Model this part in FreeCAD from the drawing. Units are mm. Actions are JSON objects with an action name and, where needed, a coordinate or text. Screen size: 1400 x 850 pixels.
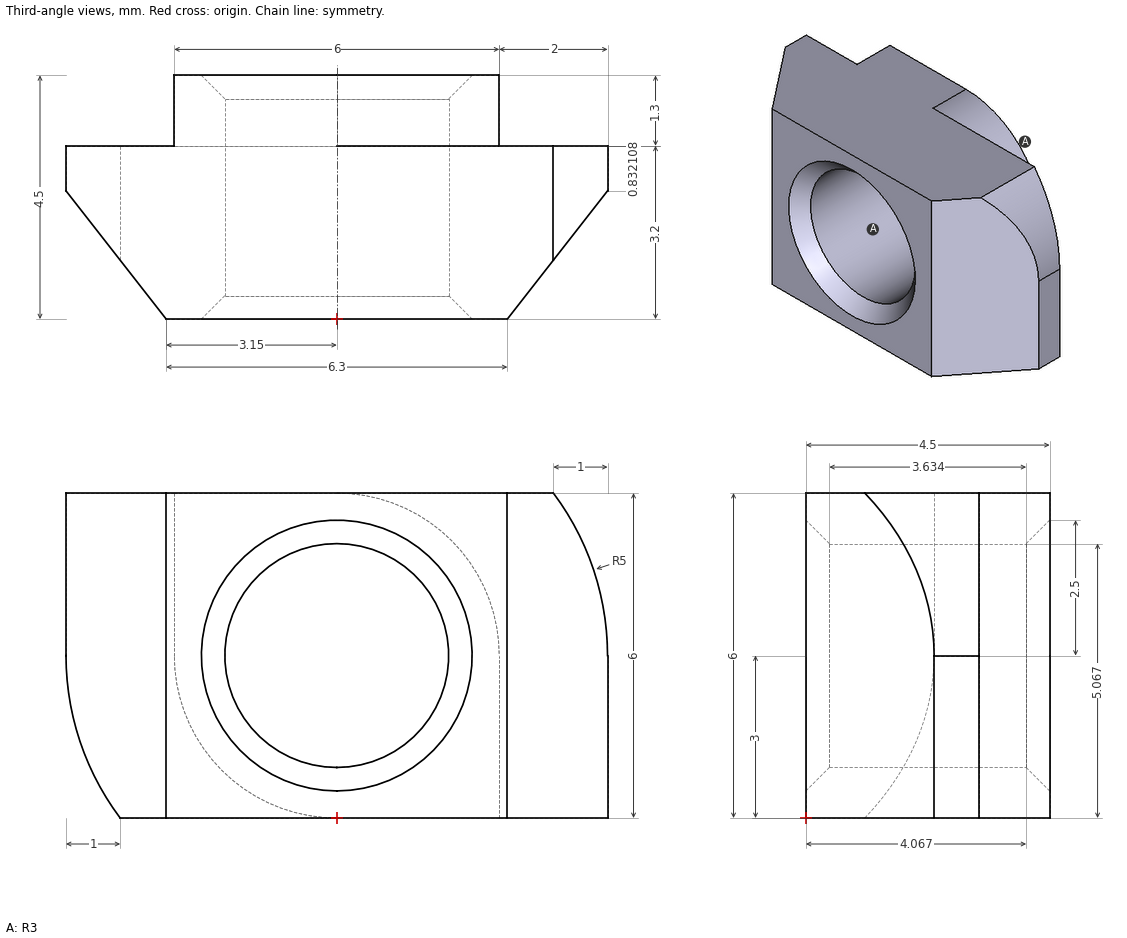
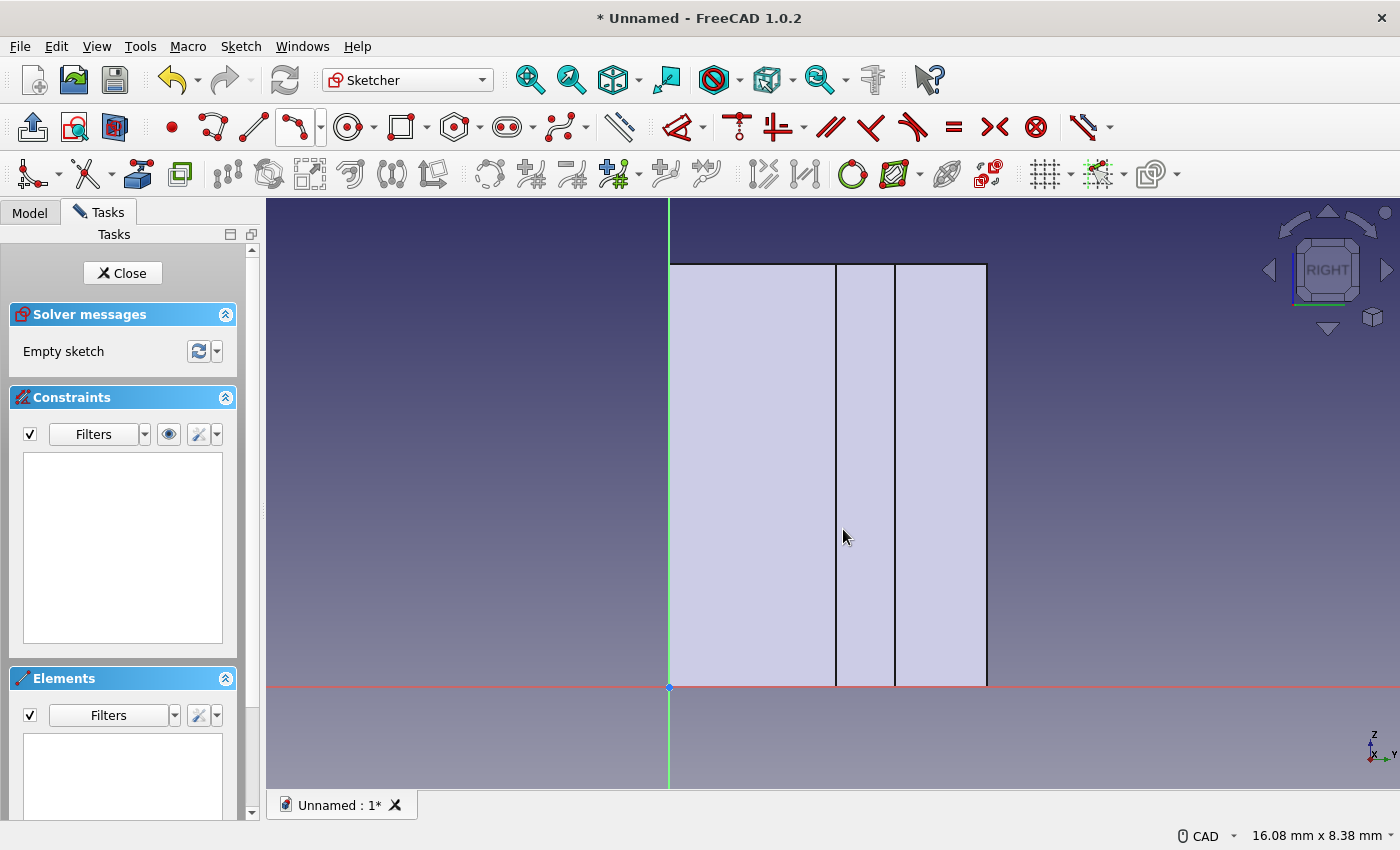
{"action": "left_click", "coordinate": [213, 128]}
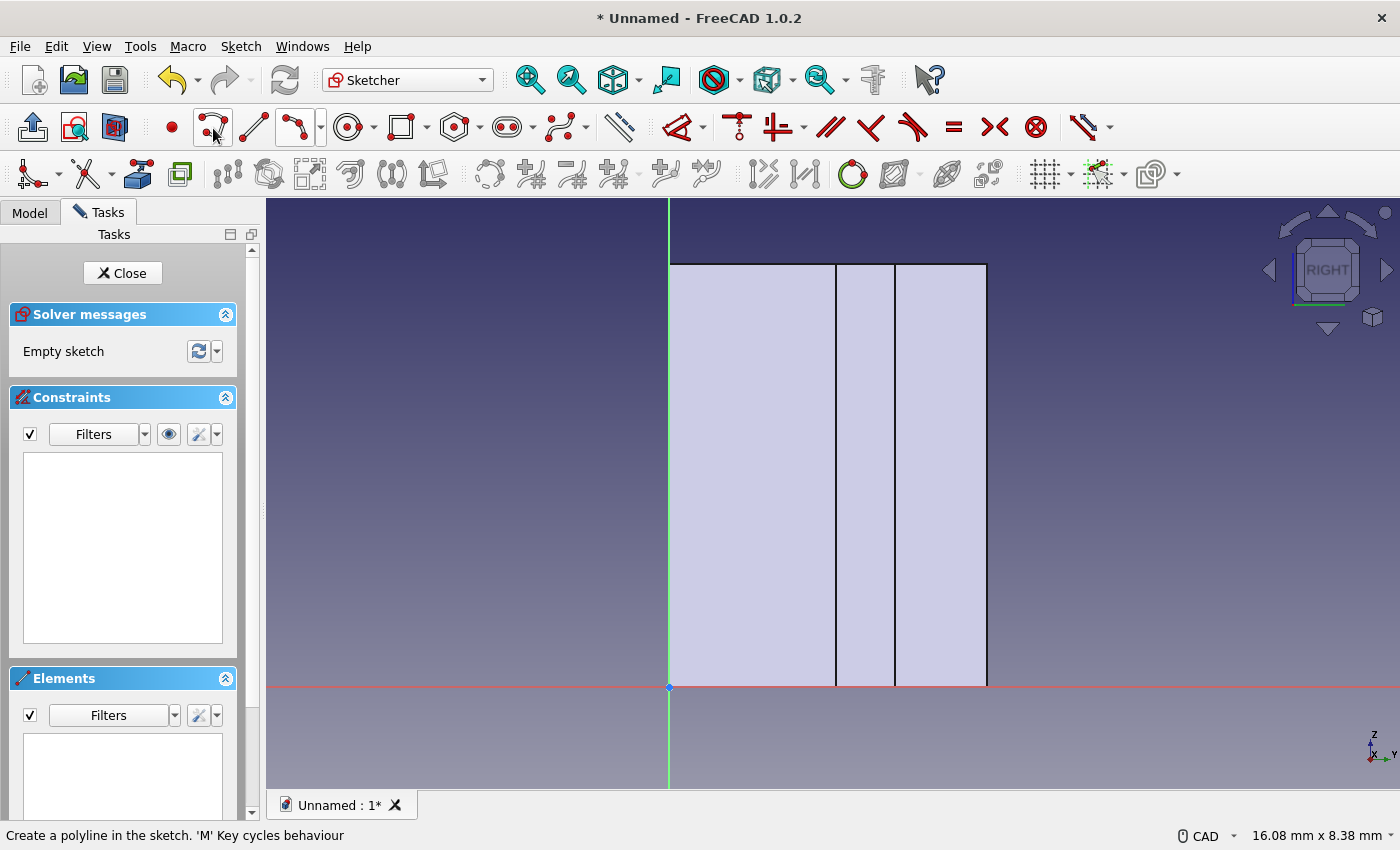
{"action": "left_click", "coordinate": [669, 476]}
{"action": "left_click", "coordinate": [987, 476]}
{"action": "left_click", "coordinate": [987, 299]}
{"action": "left_click", "coordinate": [956, 330]}
{"action": "left_click", "coordinate": [700, 330]}
{"action": "left_click", "coordinate": [678, 299]}
{"action": "left_click", "coordinate": [669, 477]}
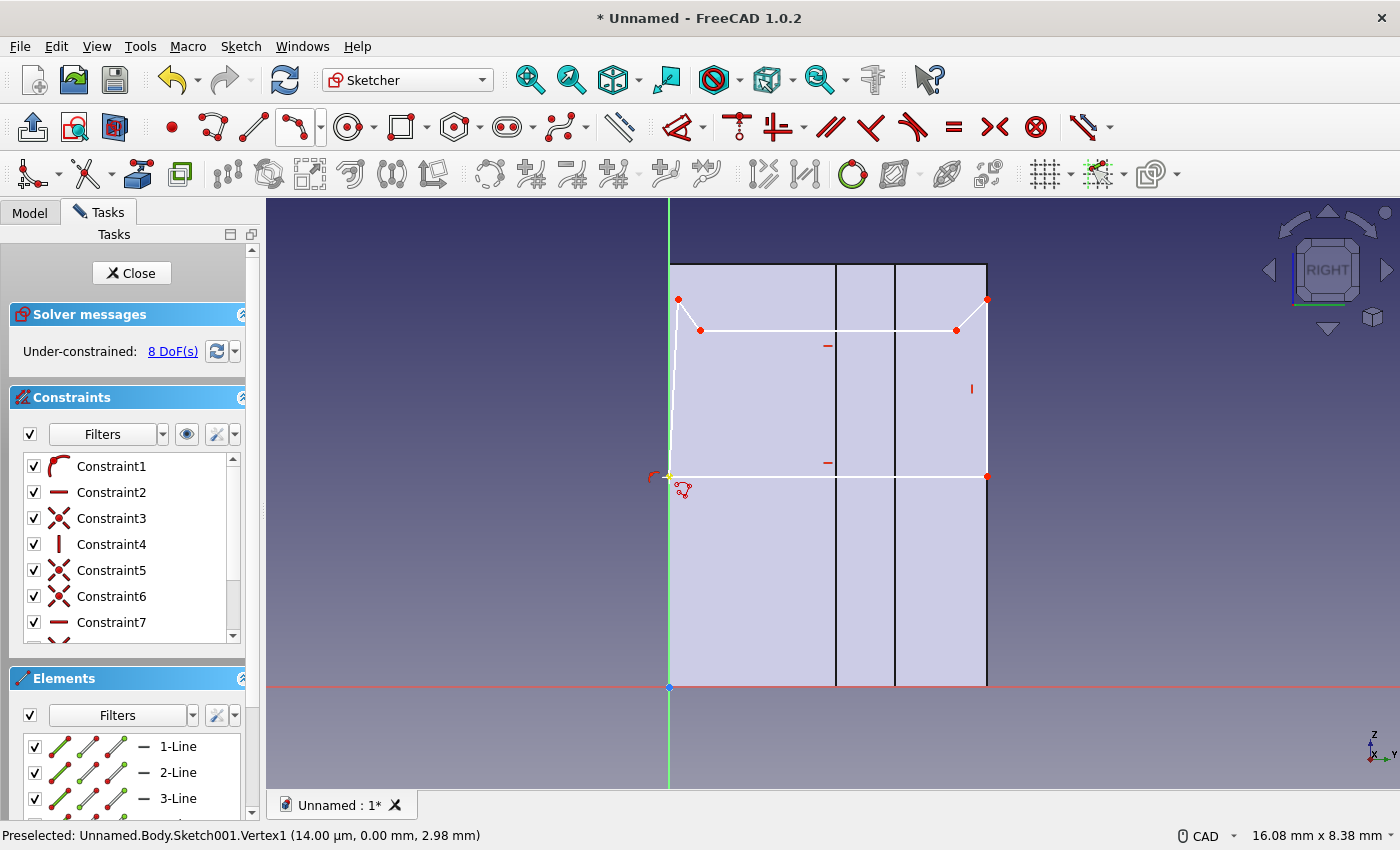
{"action": "left_click", "coordinate": [254, 128]}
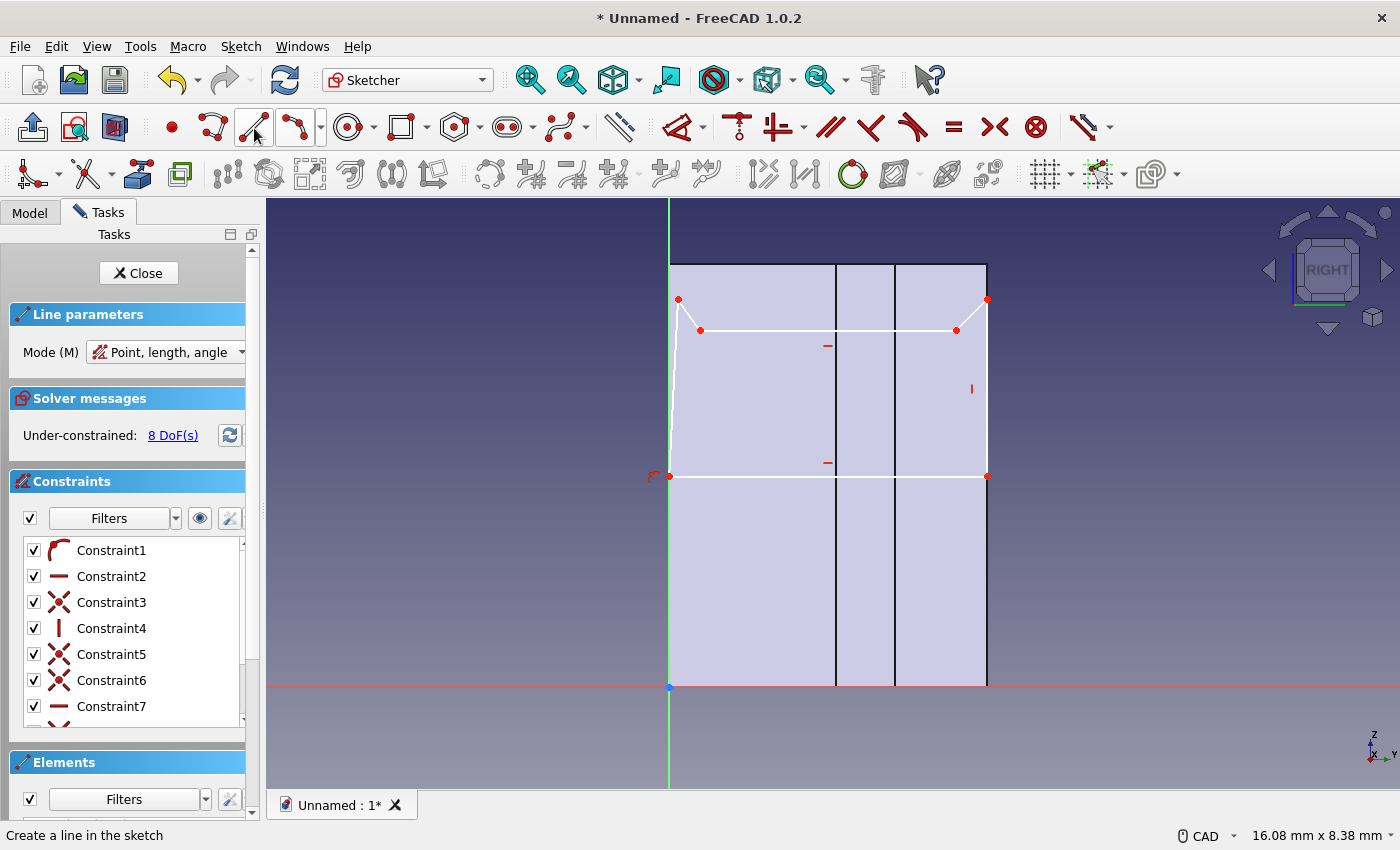
{"action": "left_click", "coordinate": [637, 476]}
{"action": "left_click", "coordinate": [542, 476]}
{"action": "key", "text": "Escape"}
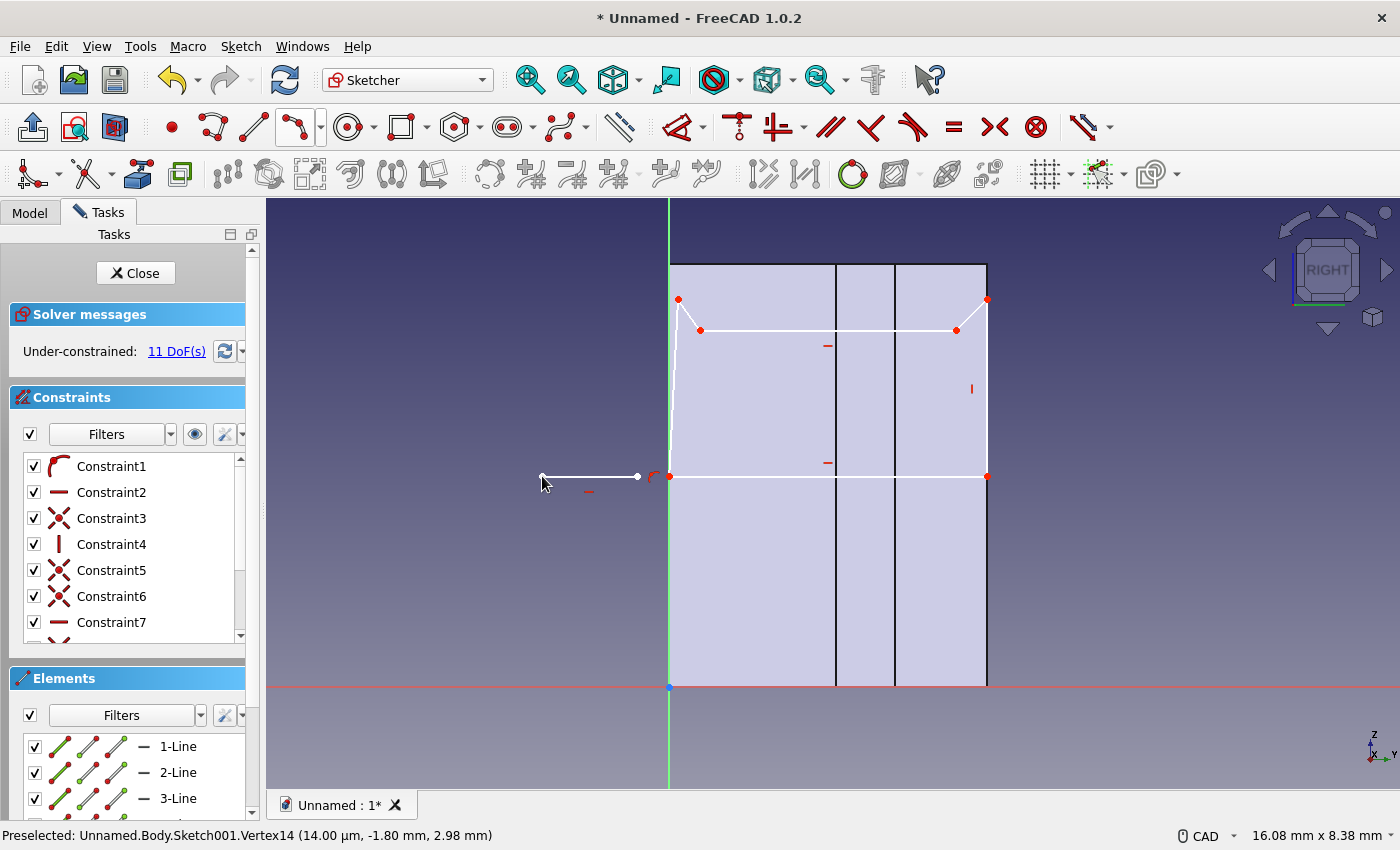
{"action": "left_click", "coordinate": [609, 477]}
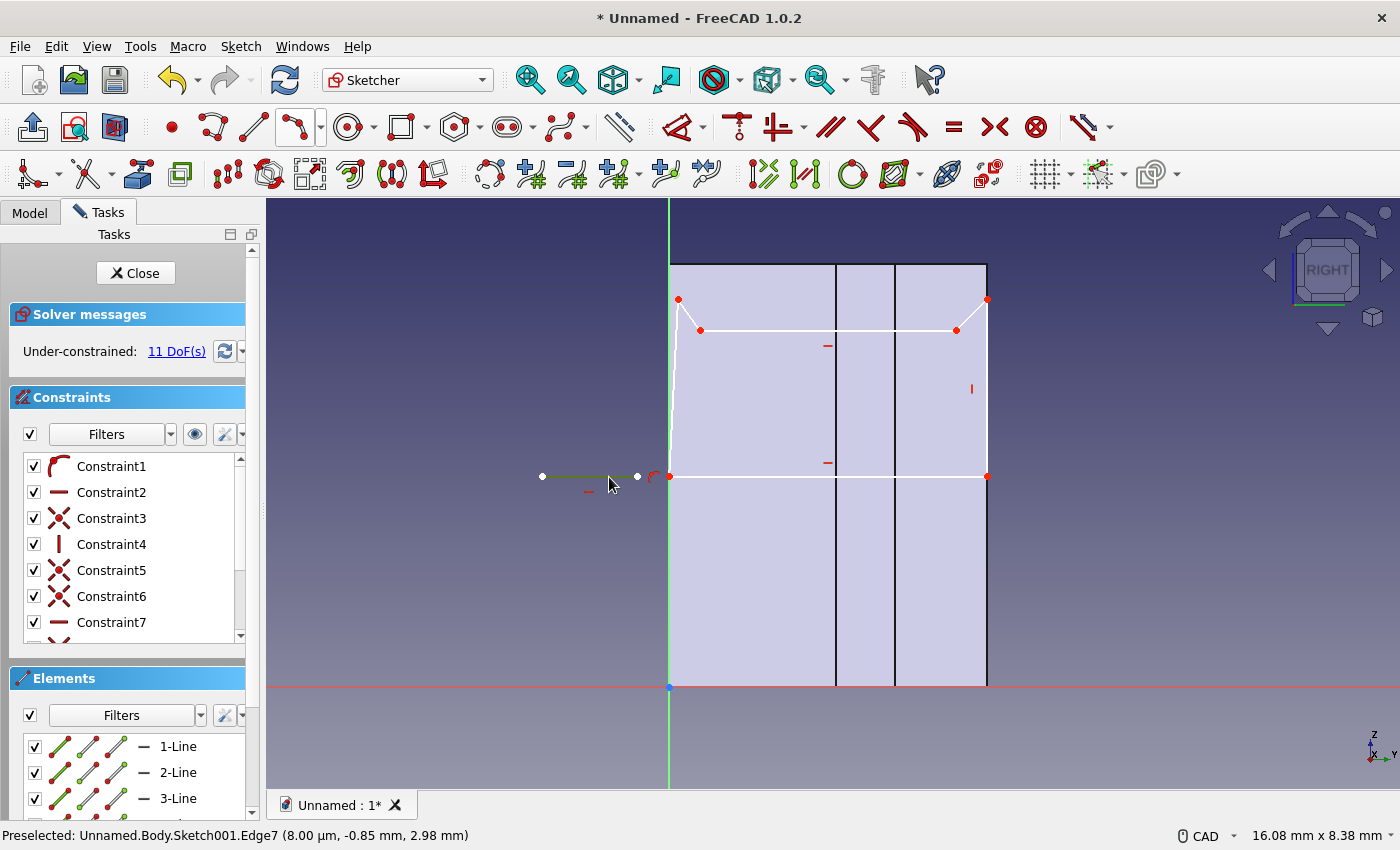
{"action": "left_click", "coordinate": [620, 128]}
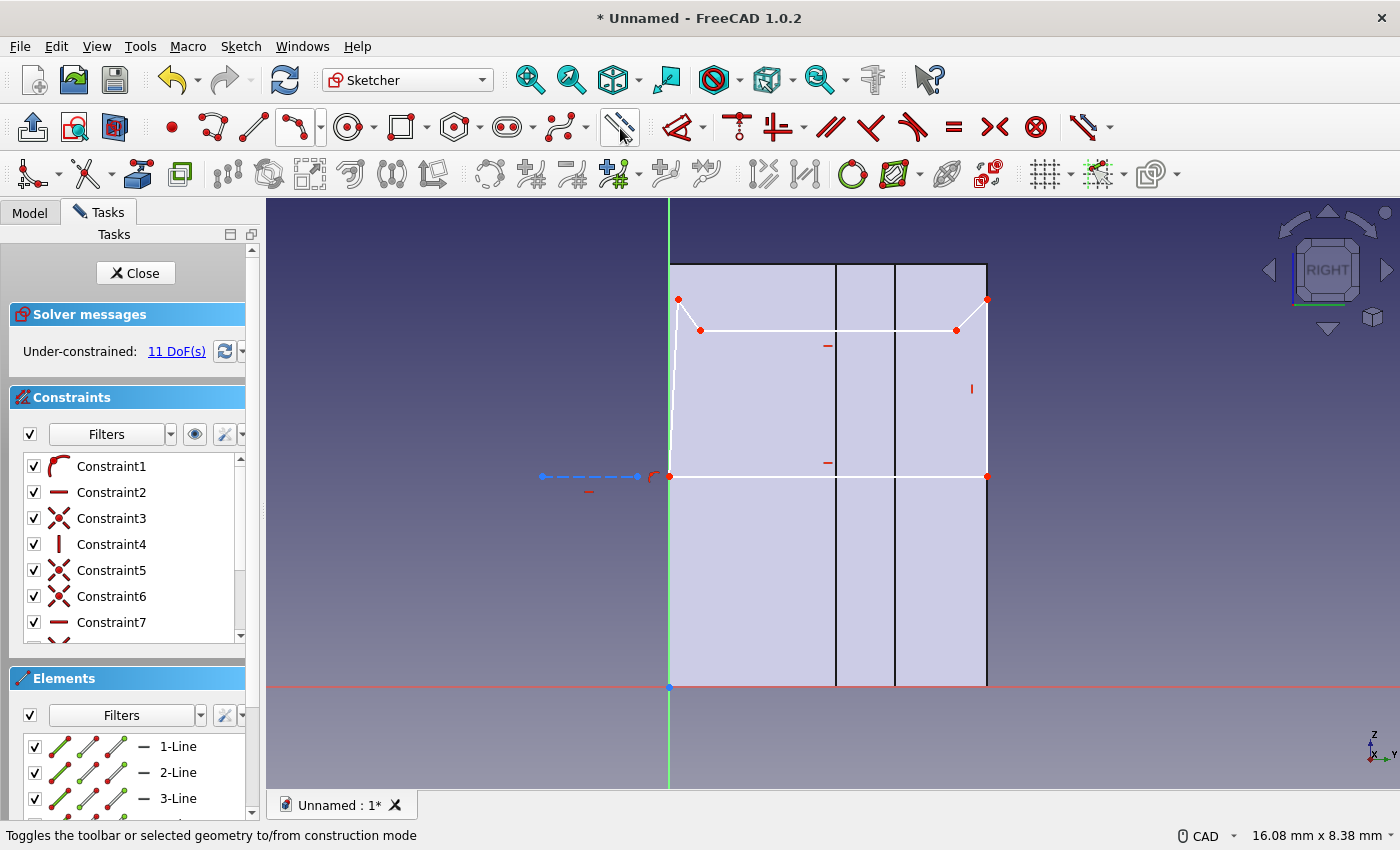
{"action": "left_click", "coordinate": [672, 424]}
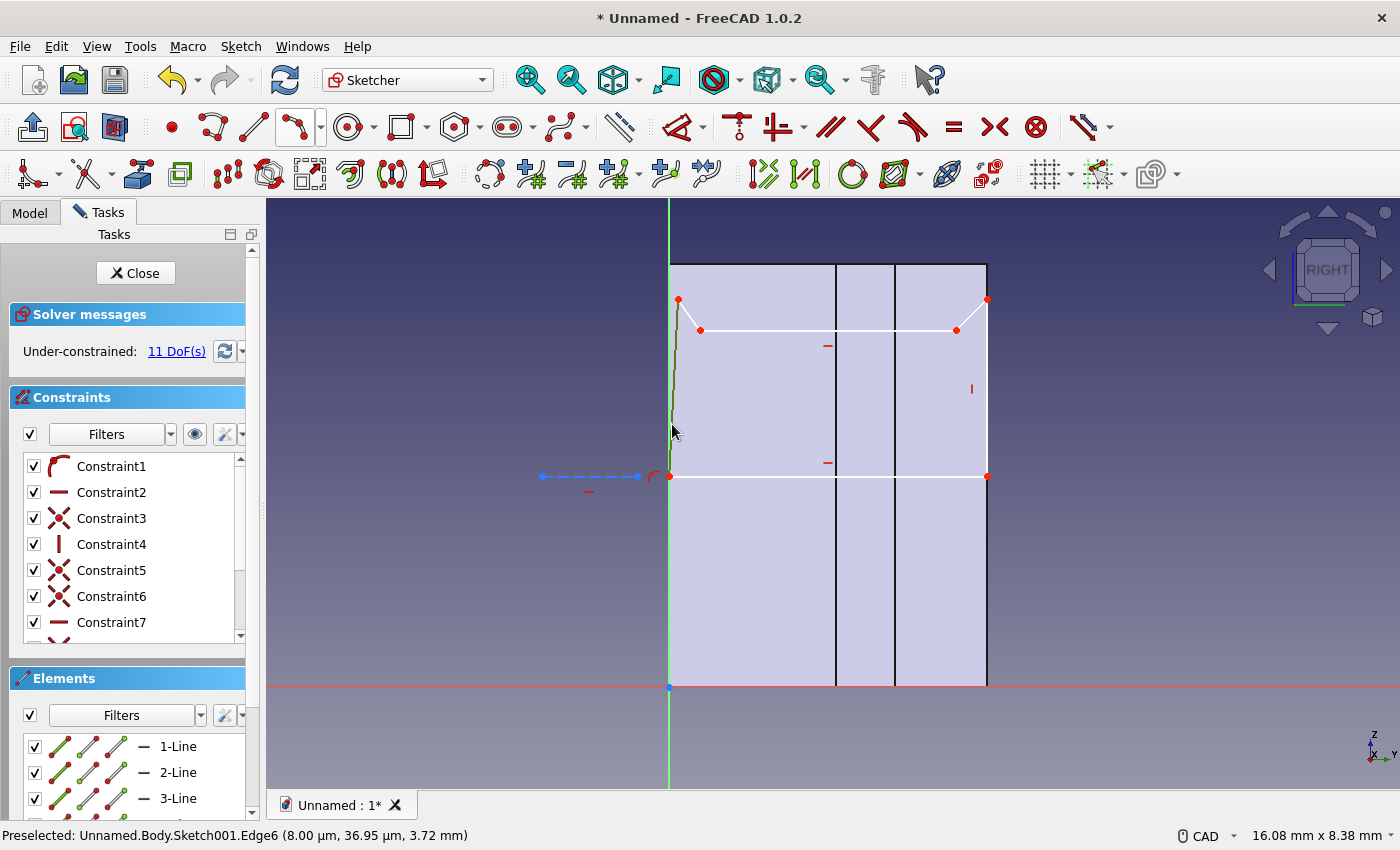
{"action": "left_click", "coordinate": [804, 128]}